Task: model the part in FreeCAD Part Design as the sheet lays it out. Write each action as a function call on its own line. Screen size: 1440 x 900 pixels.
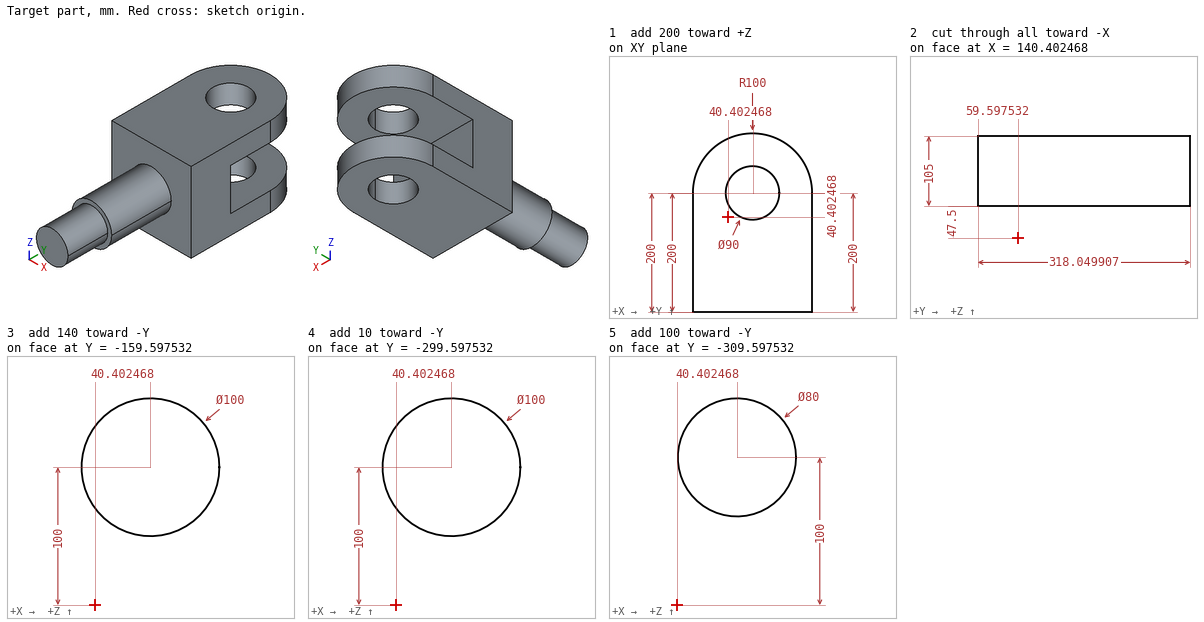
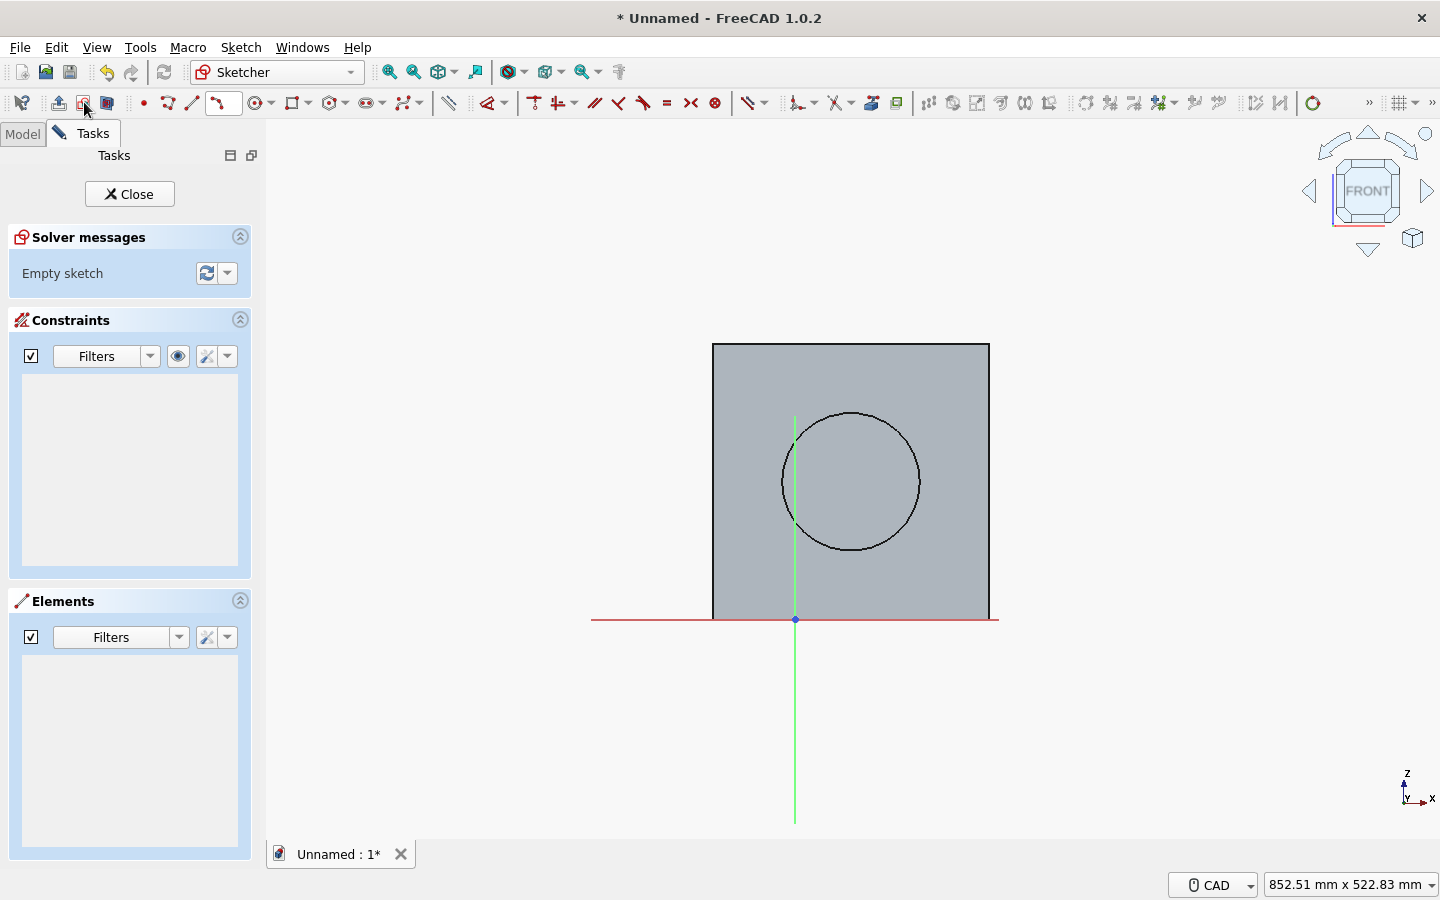
scroll(905, 559, up, 4)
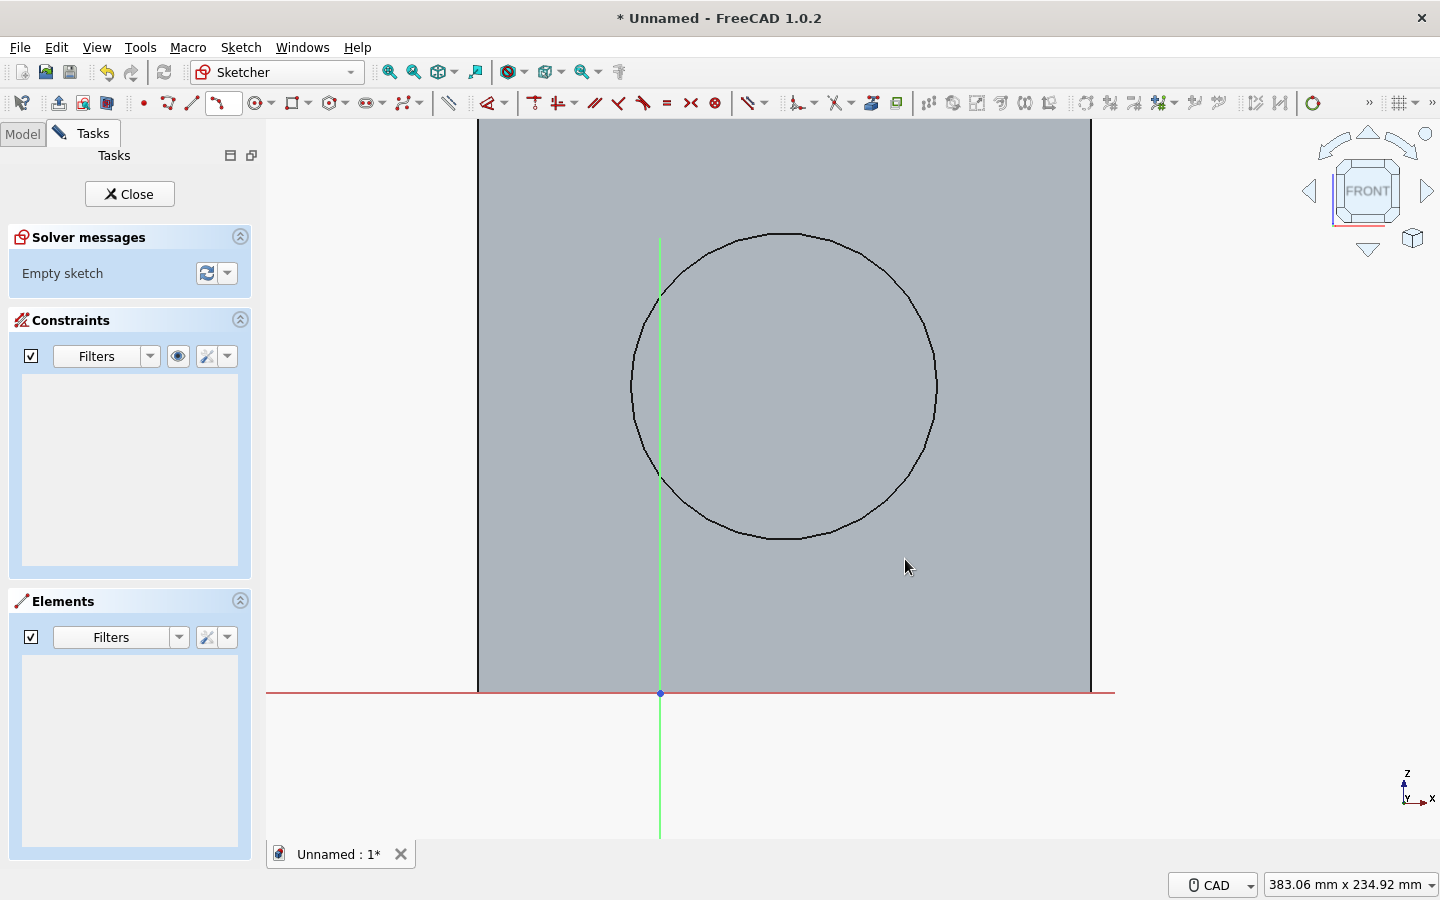
key(g)
key(c)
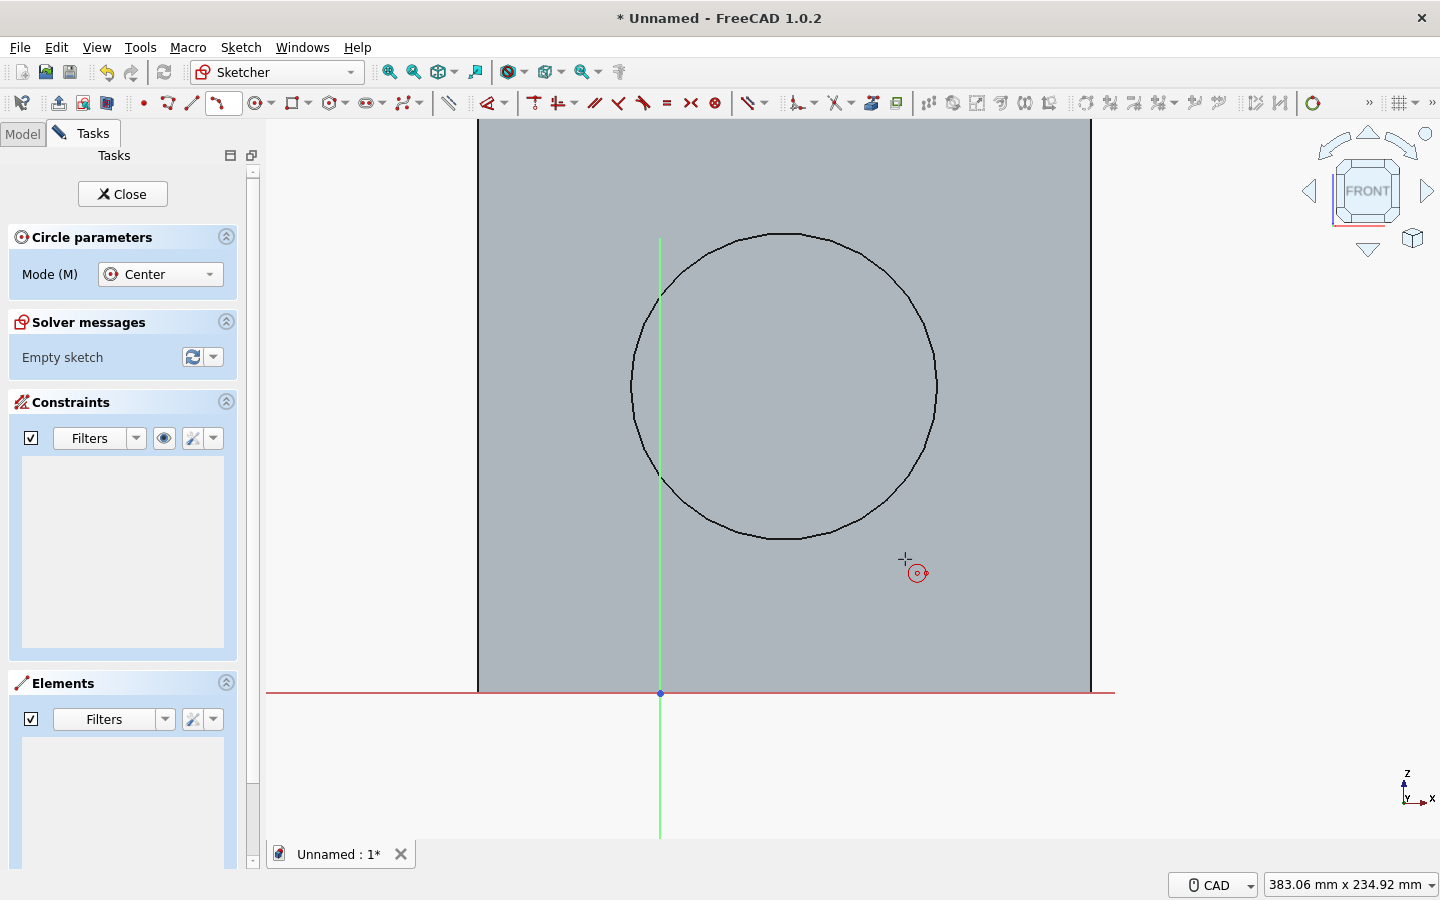
click(784, 387)
click(871, 300)
key(Escape)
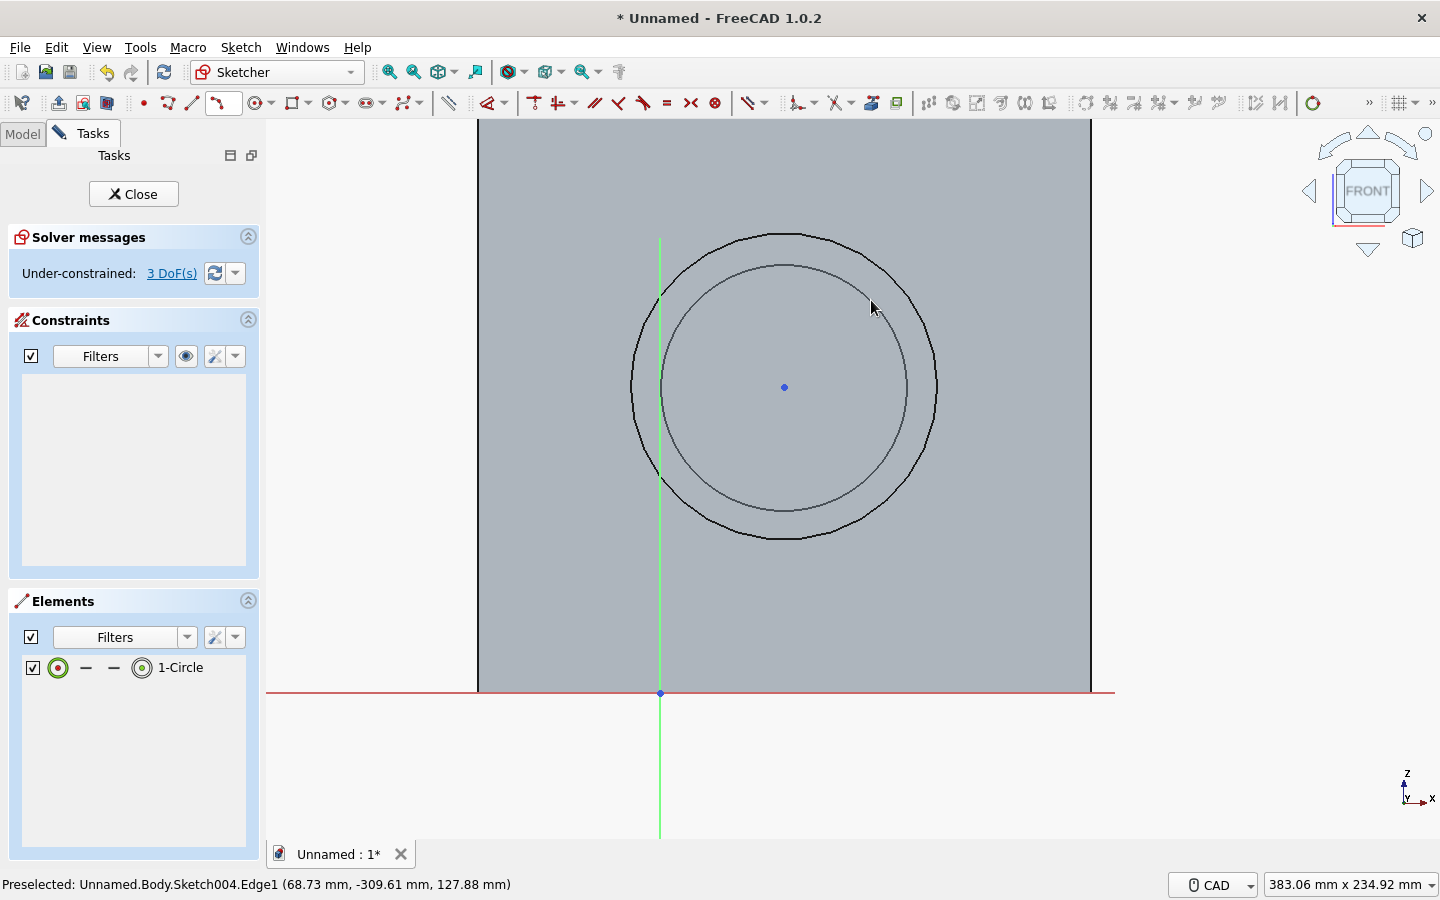
click(488, 104)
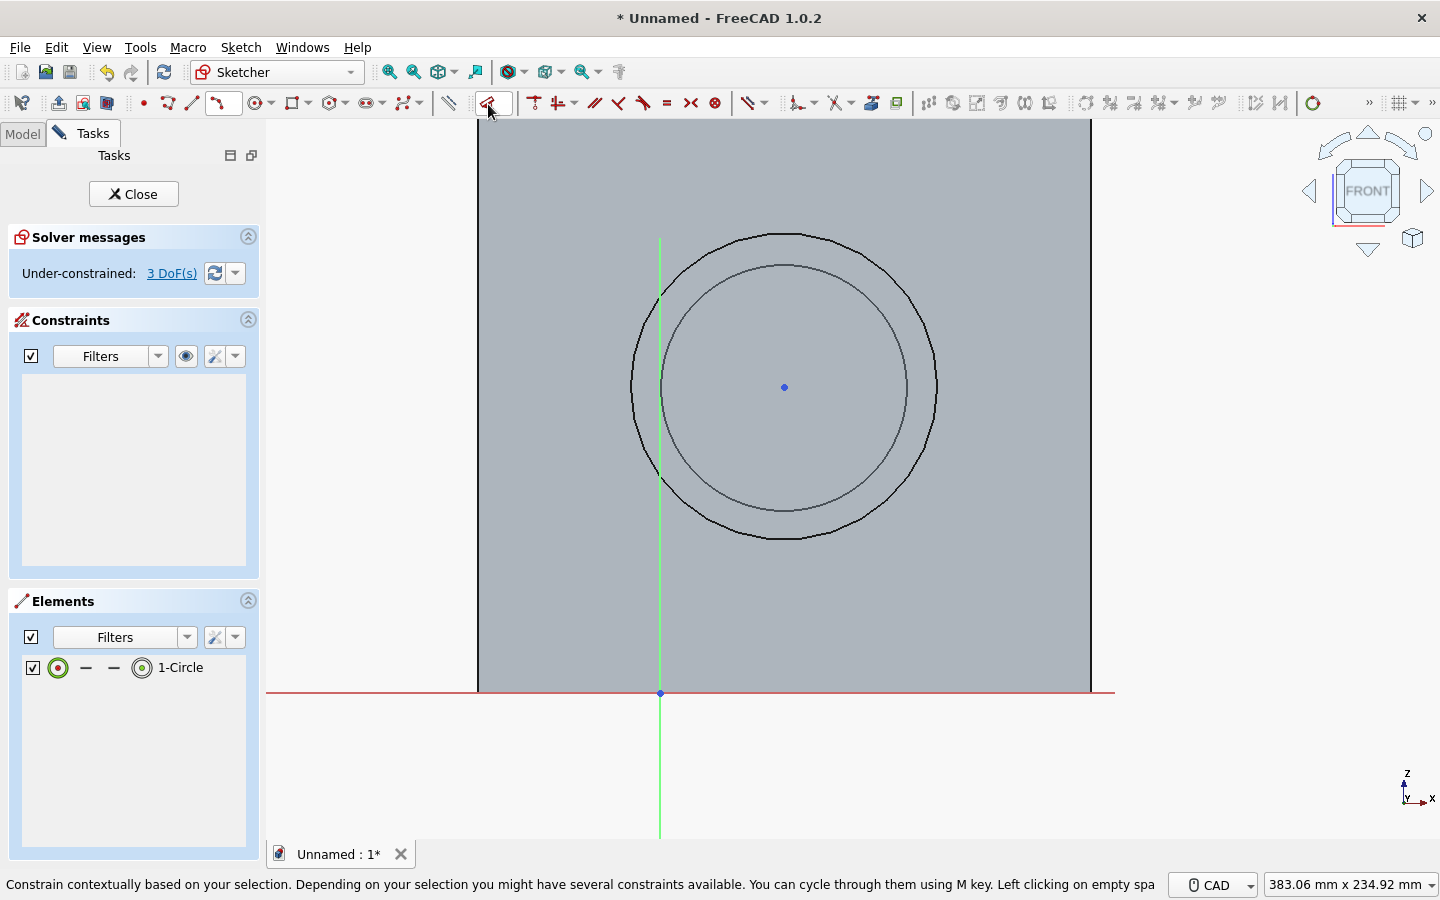
click(871, 301)
click(894, 278)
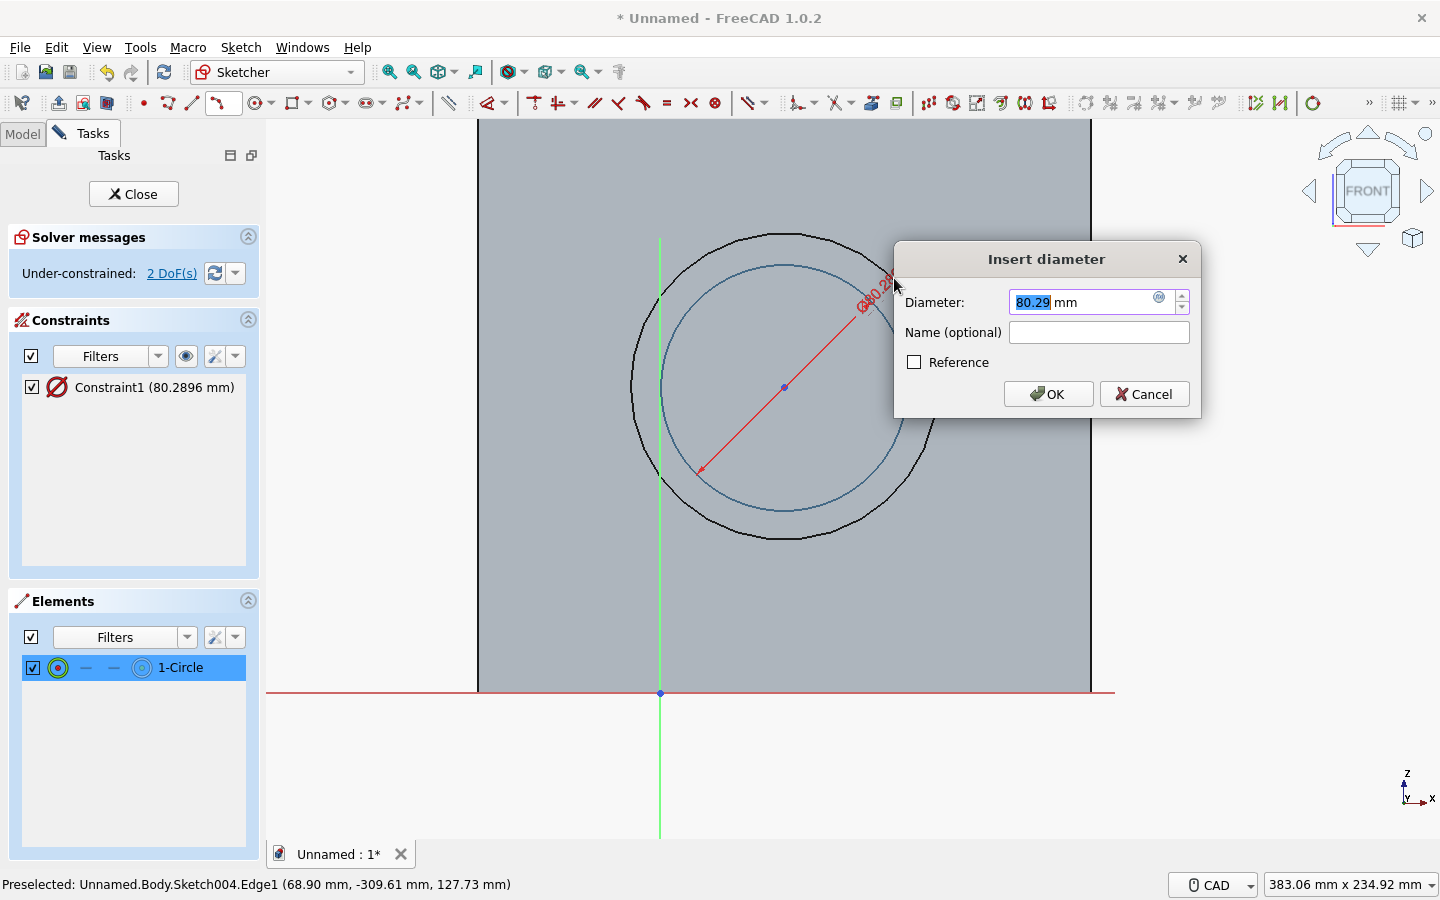
text(80)
key(Return)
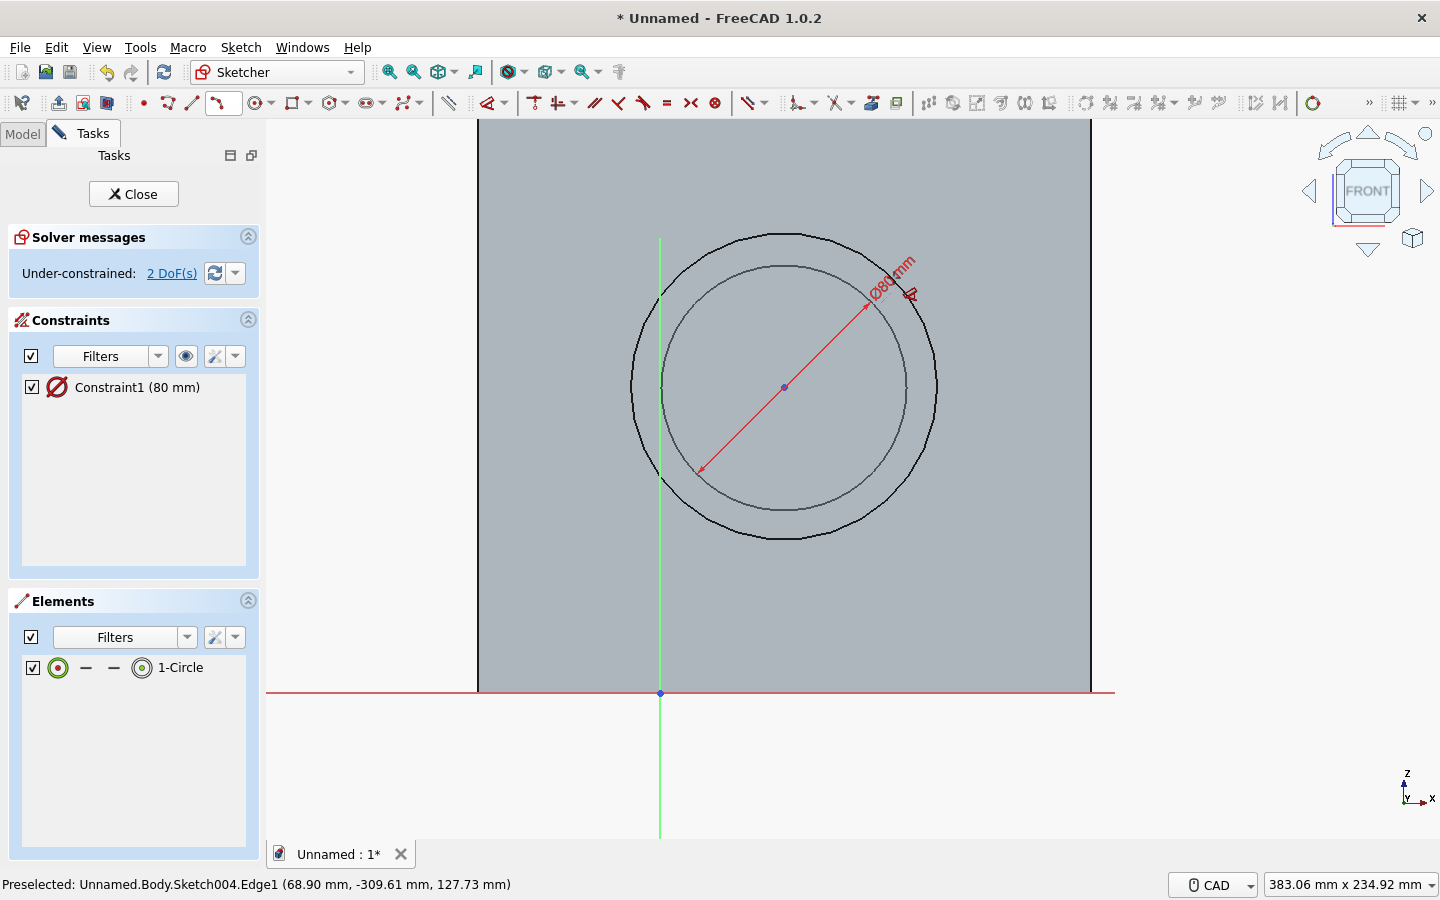
click(784, 388)
click(626, 541)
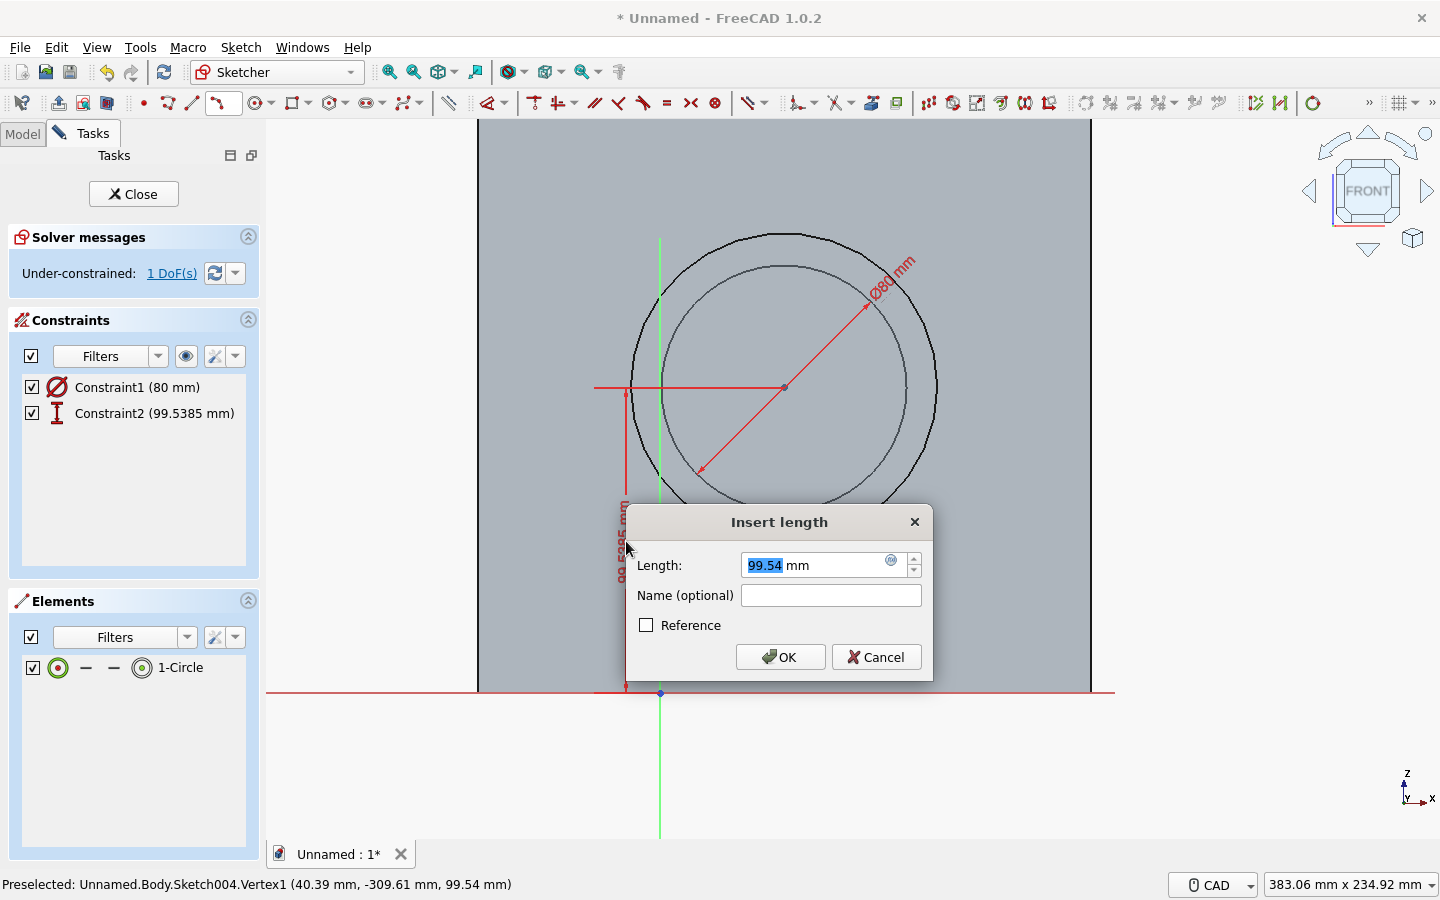
text(100)
key(Return)